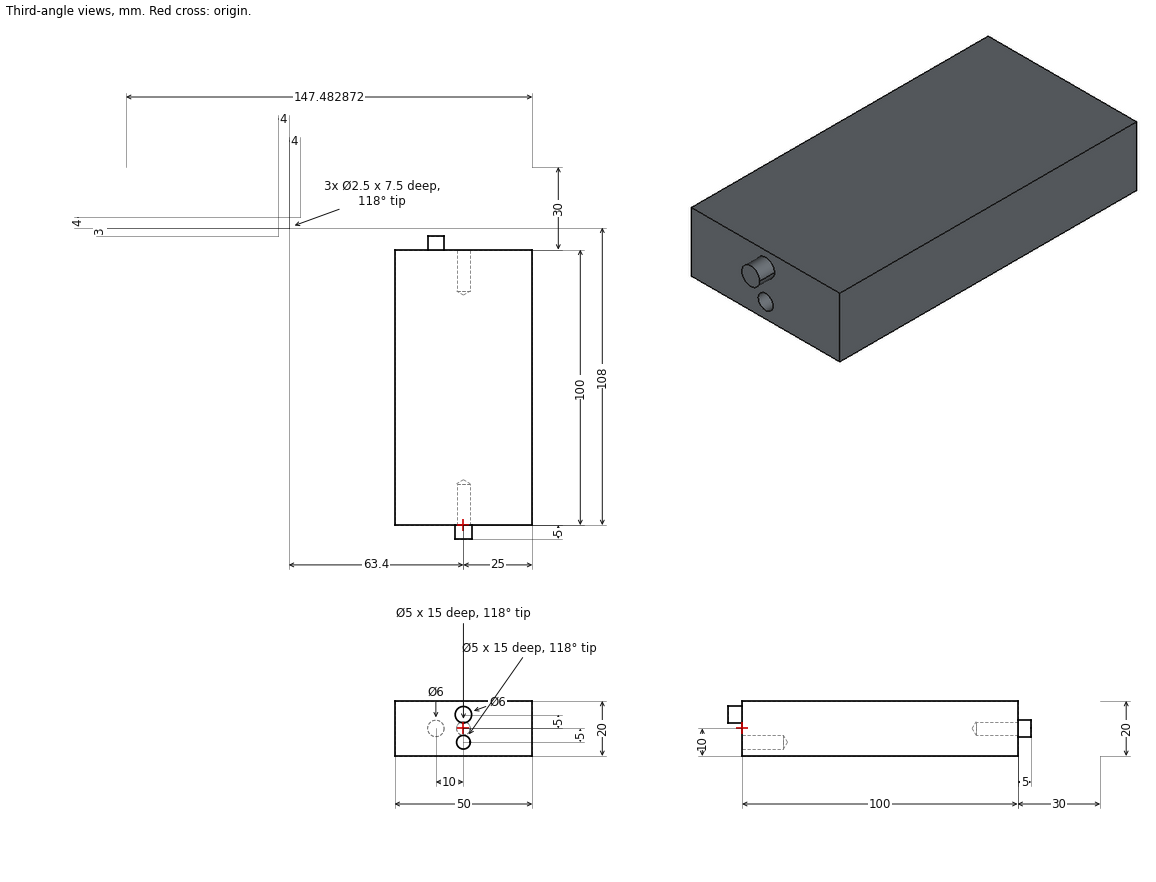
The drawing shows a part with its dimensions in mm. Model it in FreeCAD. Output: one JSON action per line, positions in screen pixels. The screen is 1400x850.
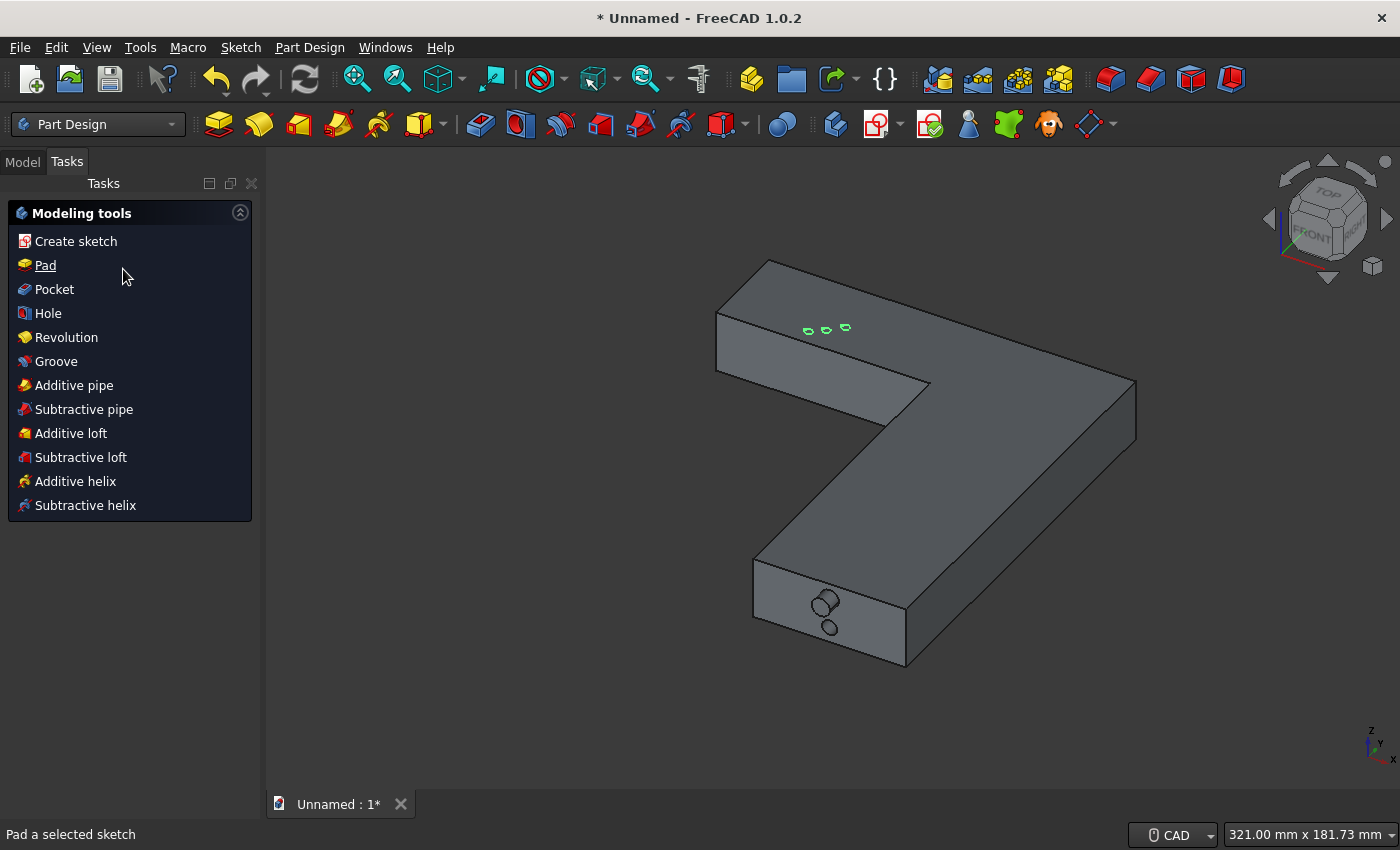
{"action": "left_click", "coordinate": [522, 124]}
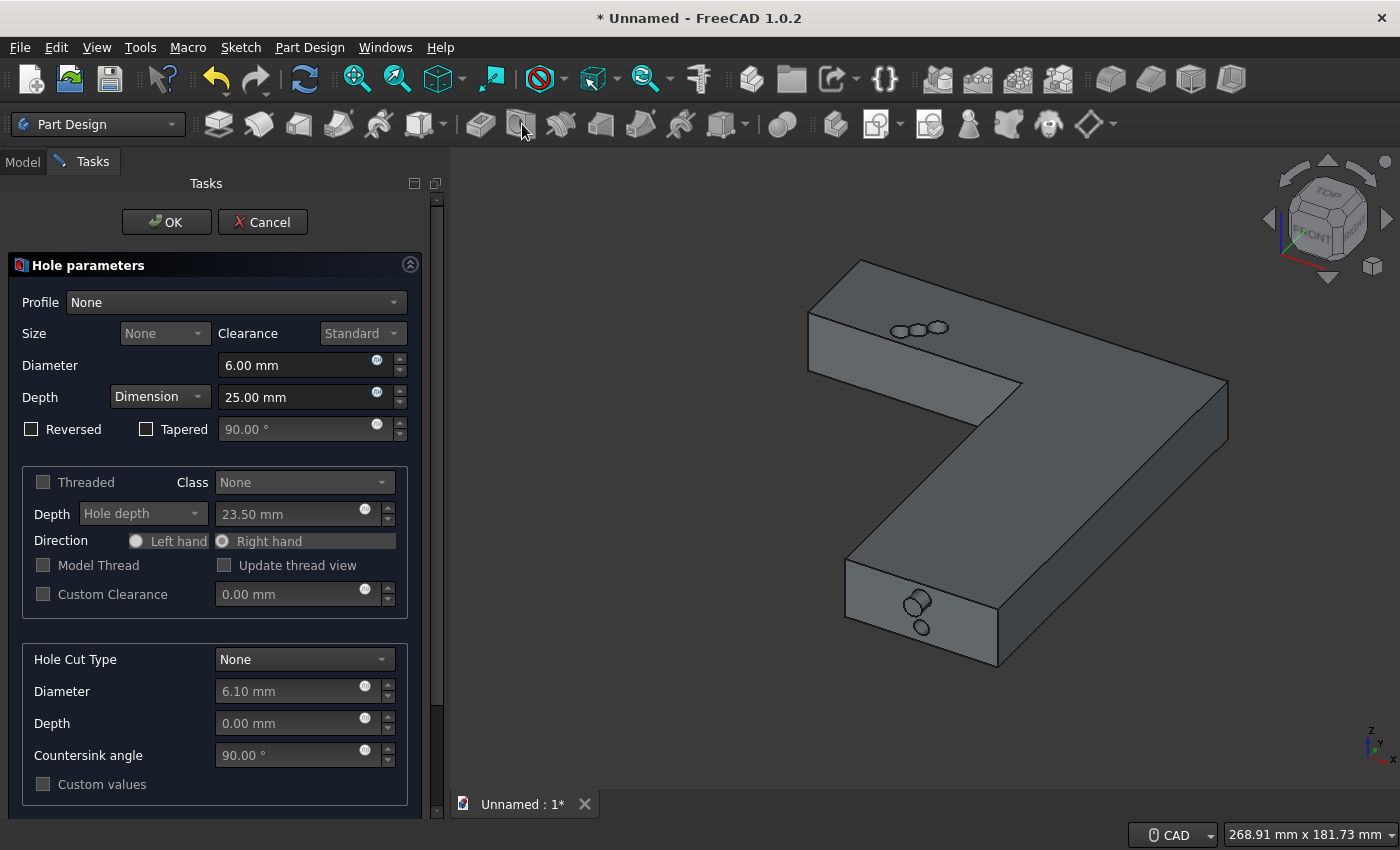
{"action": "triple_click", "coordinate": [305, 365]}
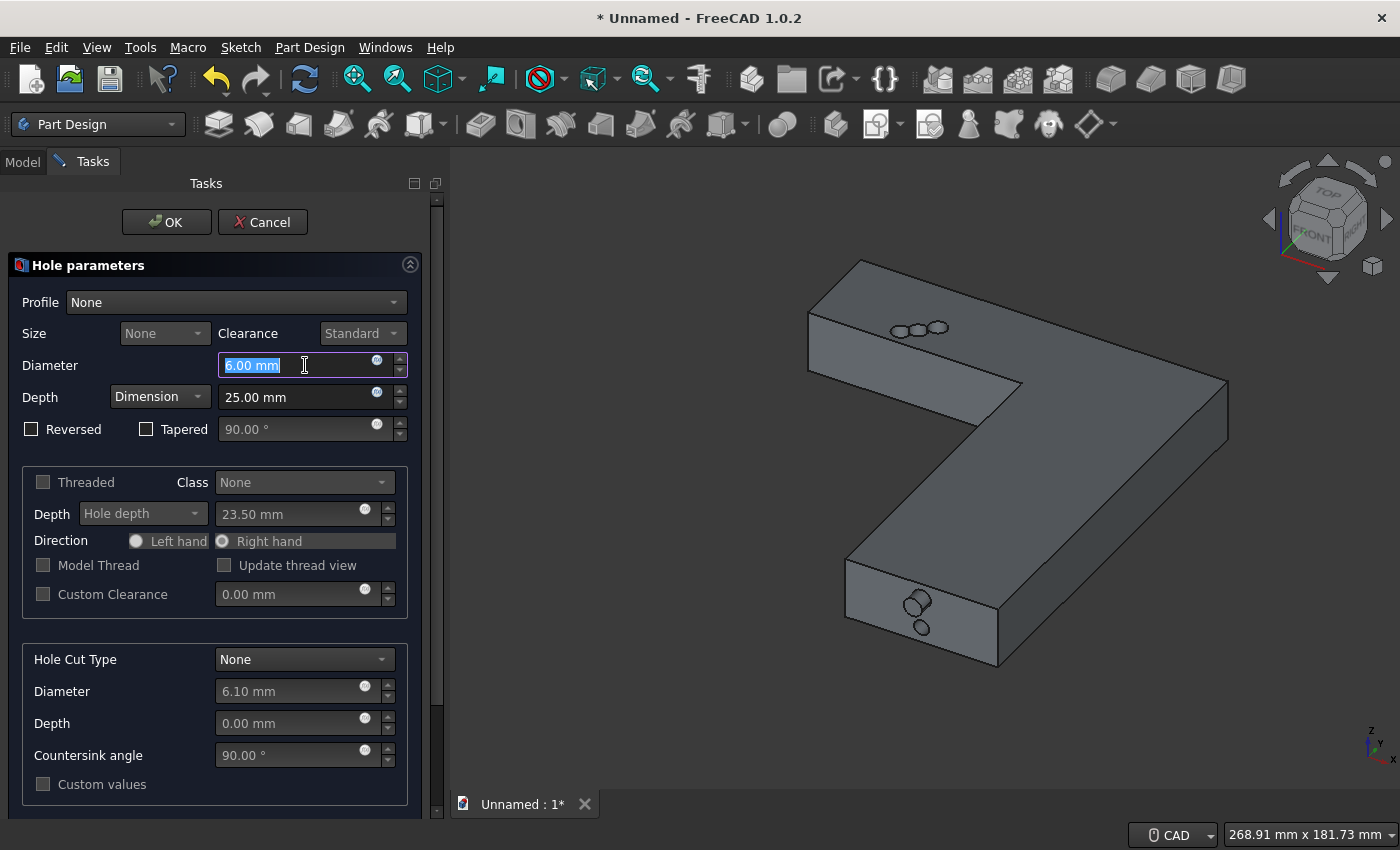
{"action": "type", "text": "2.5"}
{"action": "key", "text": "Tab"}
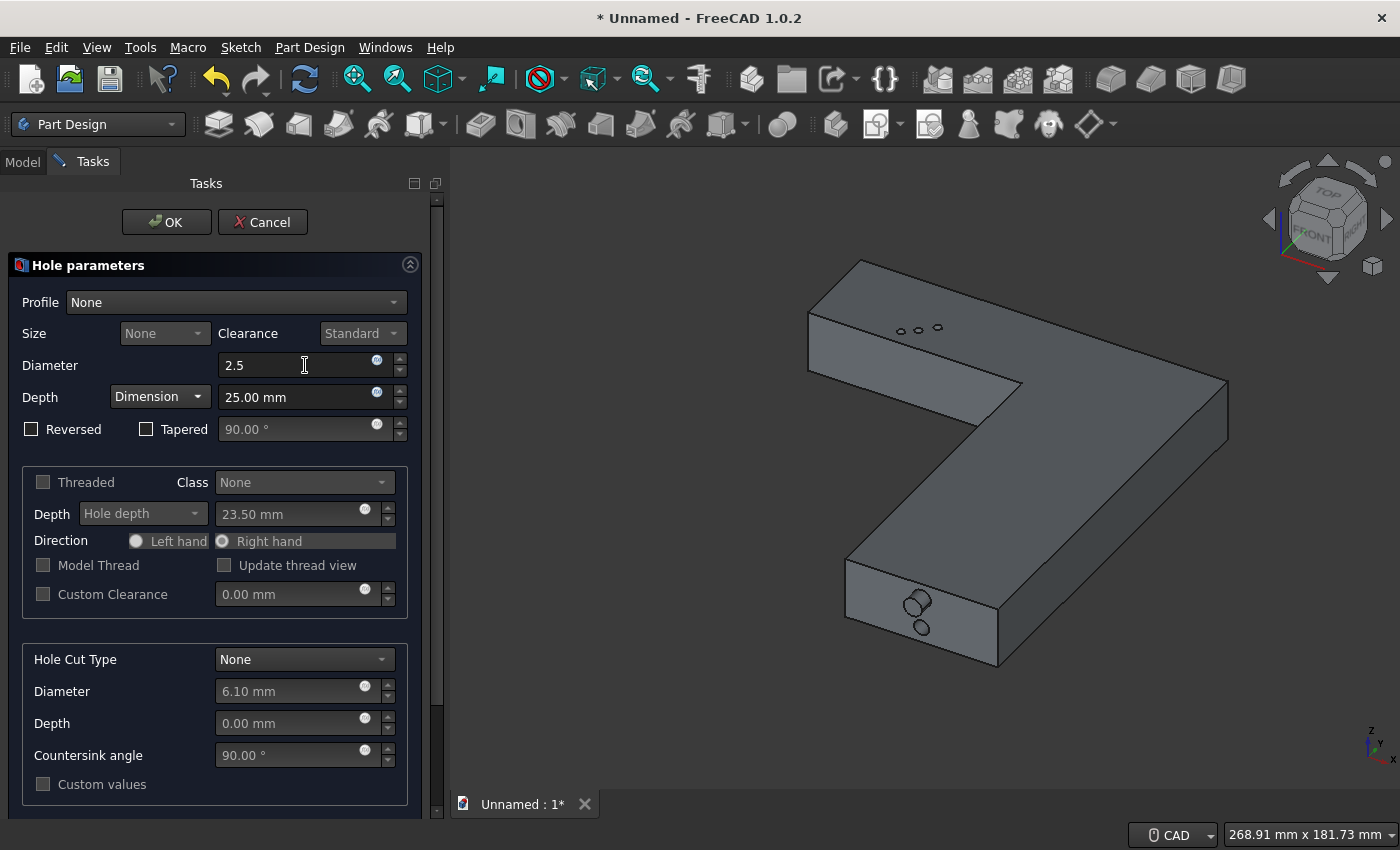
{"action": "triple_click", "coordinate": [305, 397]}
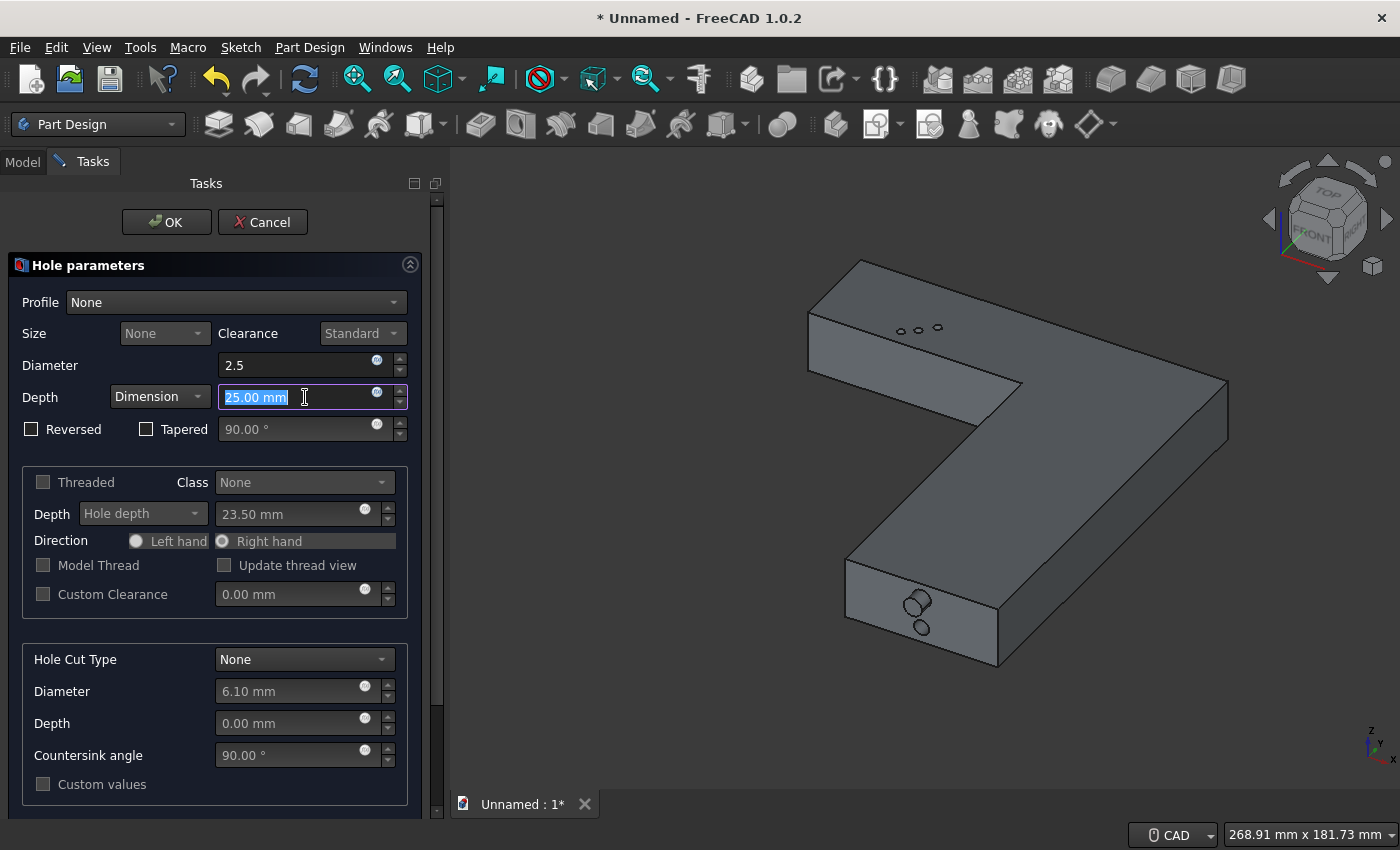
{"action": "type", "text": "7.5"}
{"action": "key", "text": "Tab"}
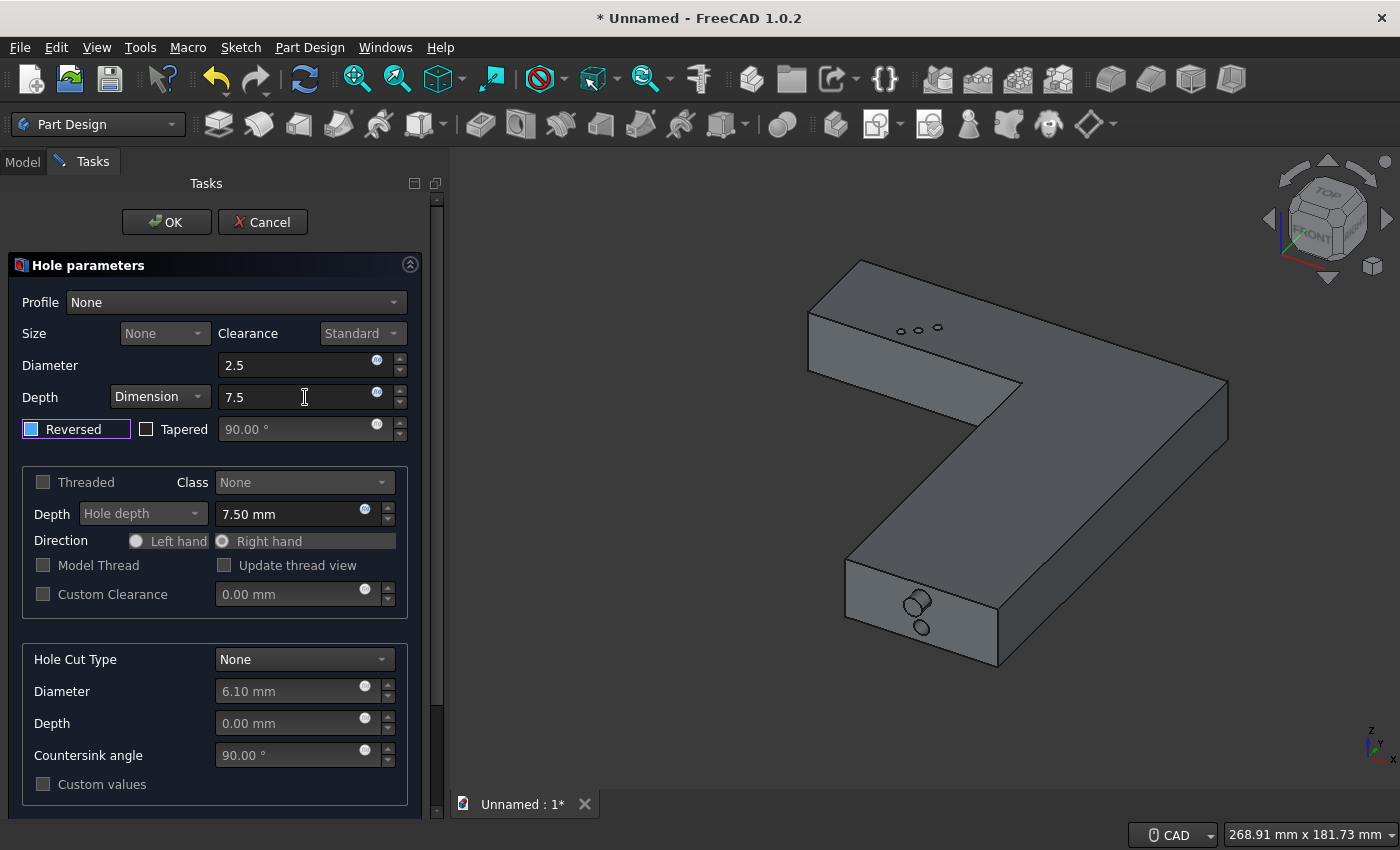
{"action": "left_click", "coordinate": [167, 222]}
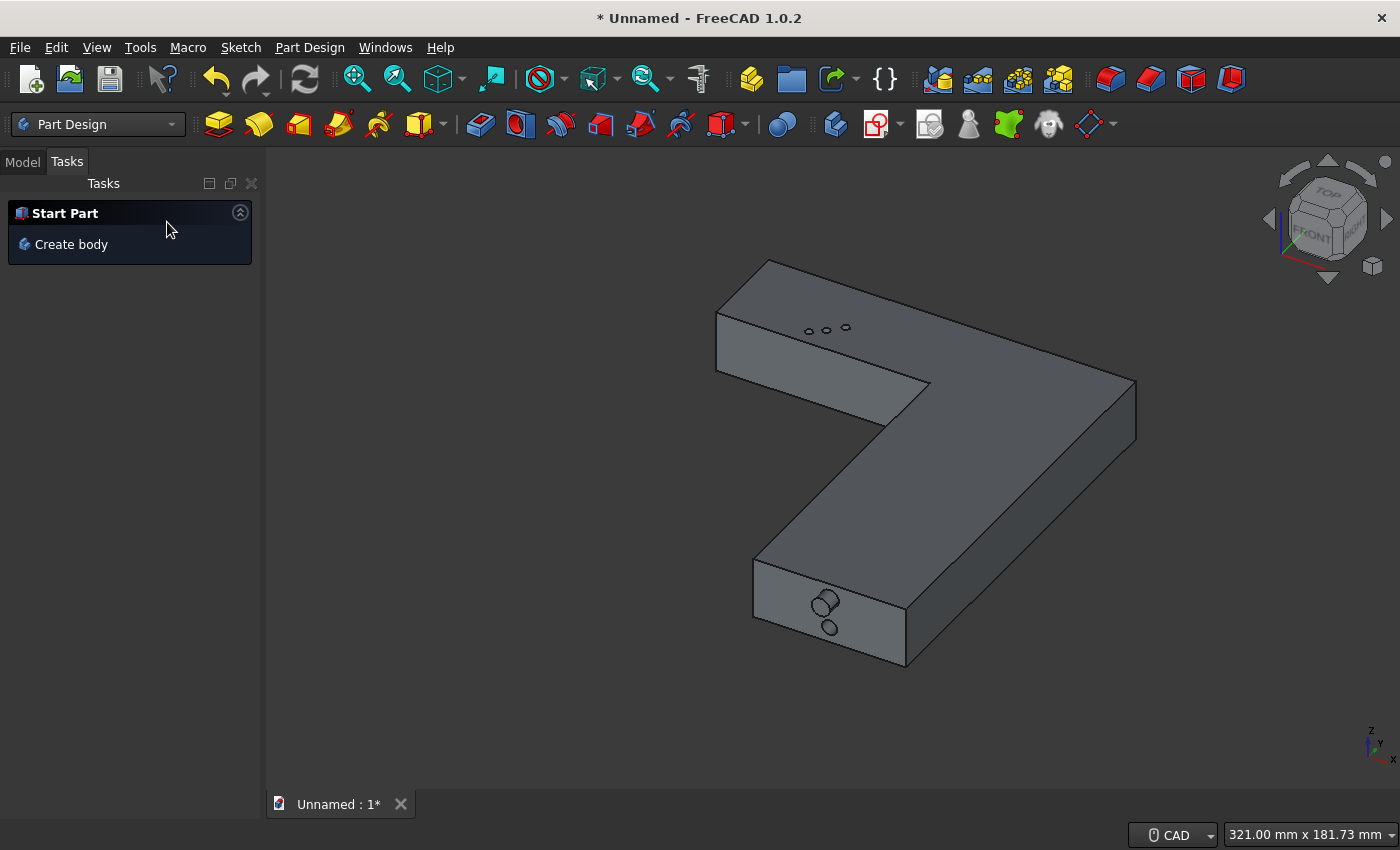
{"action": "left_click", "coordinate": [1008, 403]}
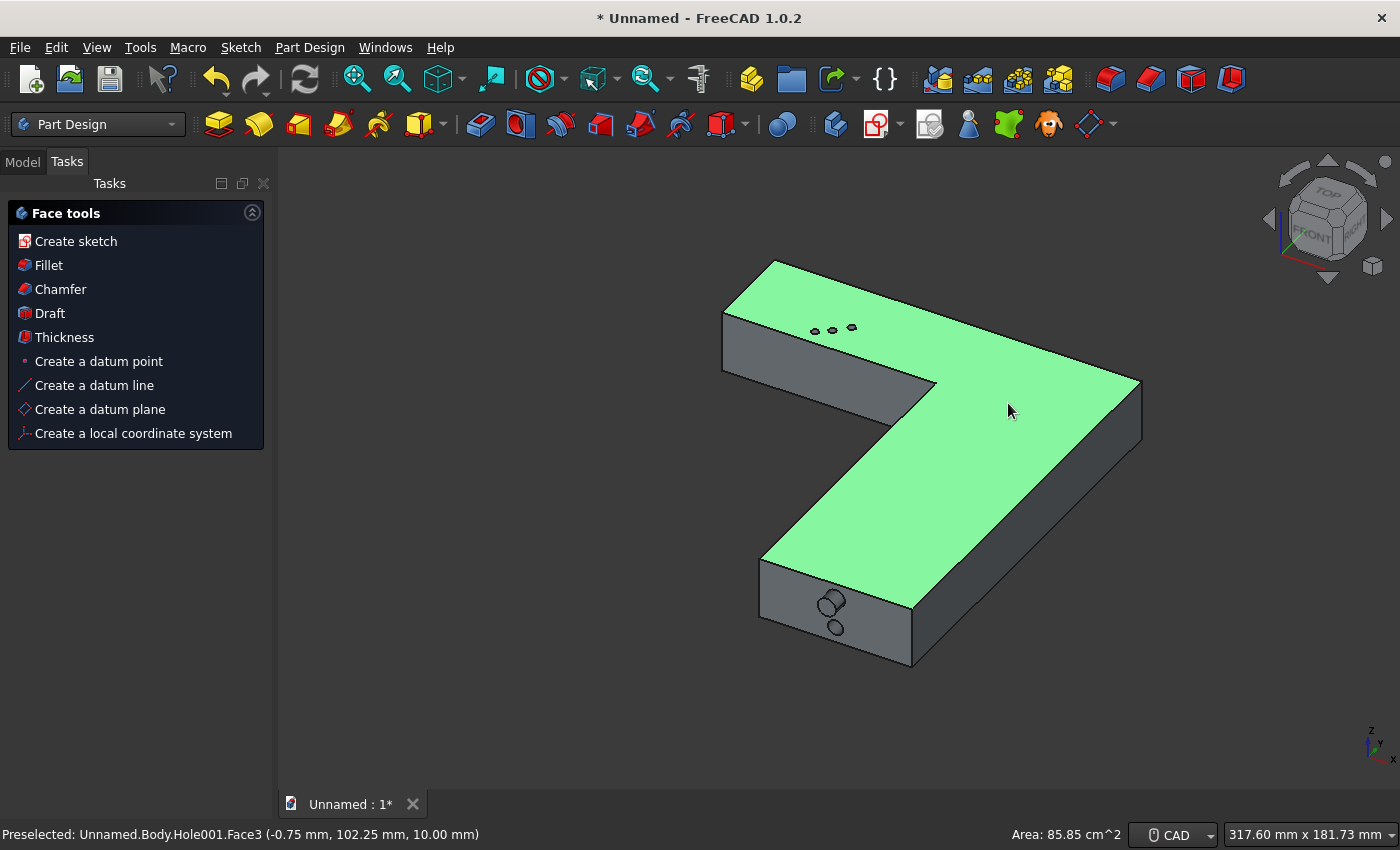
{"action": "left_click", "coordinate": [876, 124]}